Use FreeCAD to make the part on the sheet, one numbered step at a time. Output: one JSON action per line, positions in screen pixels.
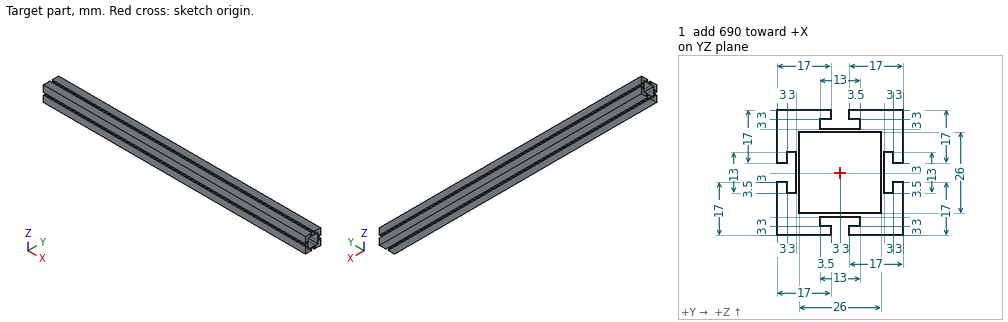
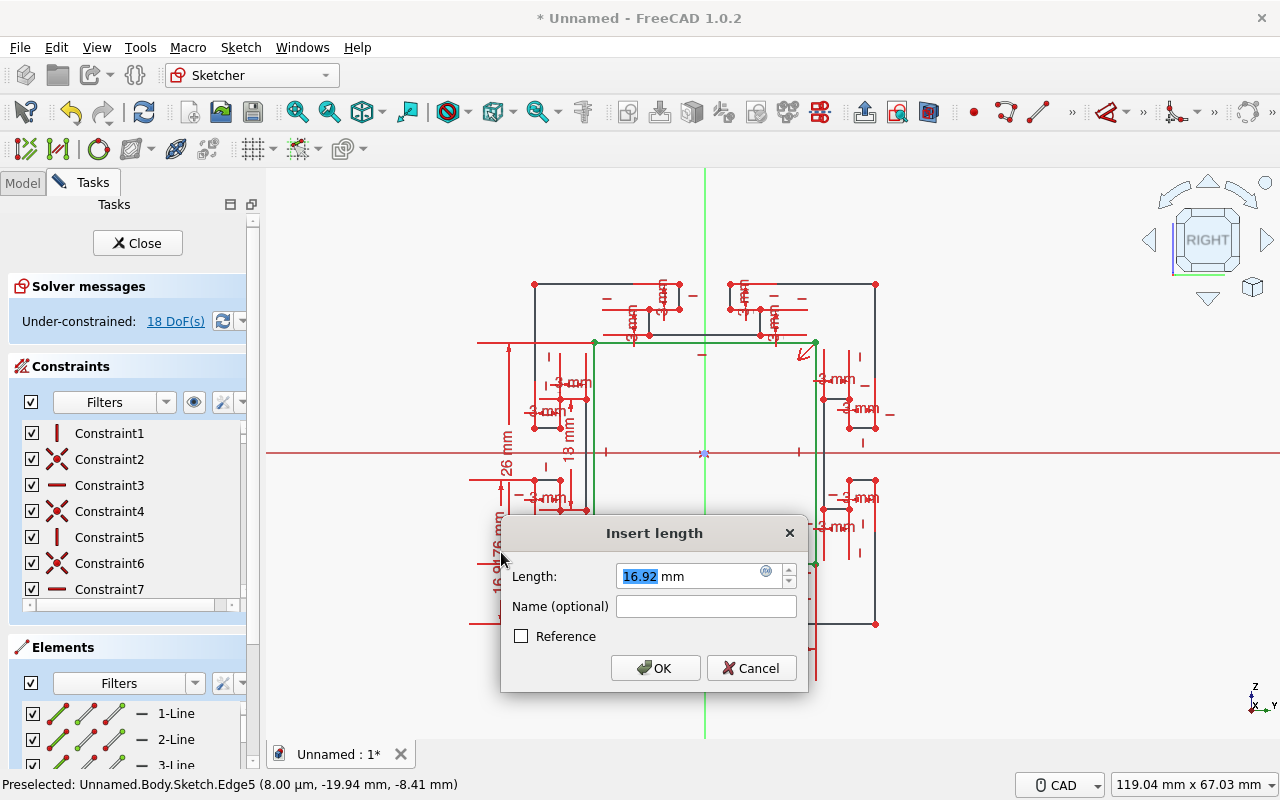
{"action": "type", "text": "17"}
{"action": "key", "text": "Return"}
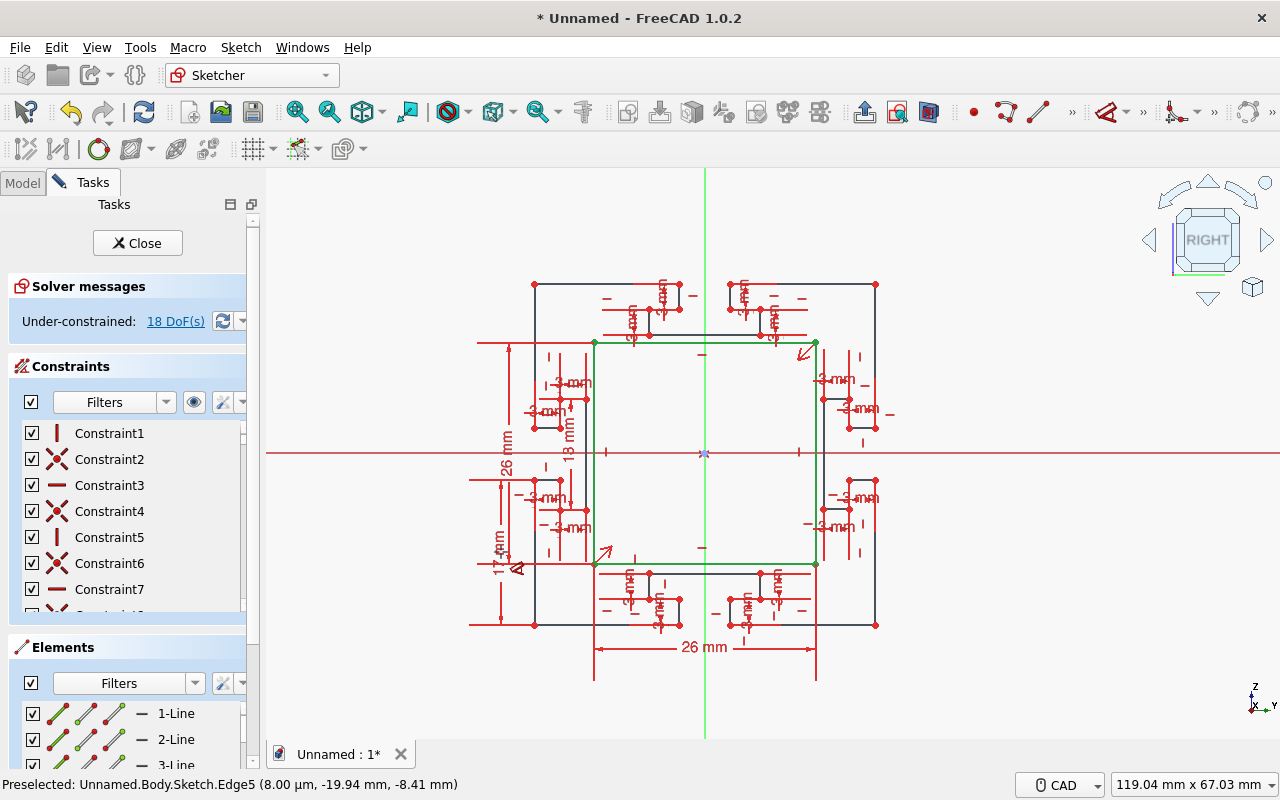
{"action": "left_click", "coordinate": [578, 625]}
{"action": "left_click", "coordinate": [607, 659]}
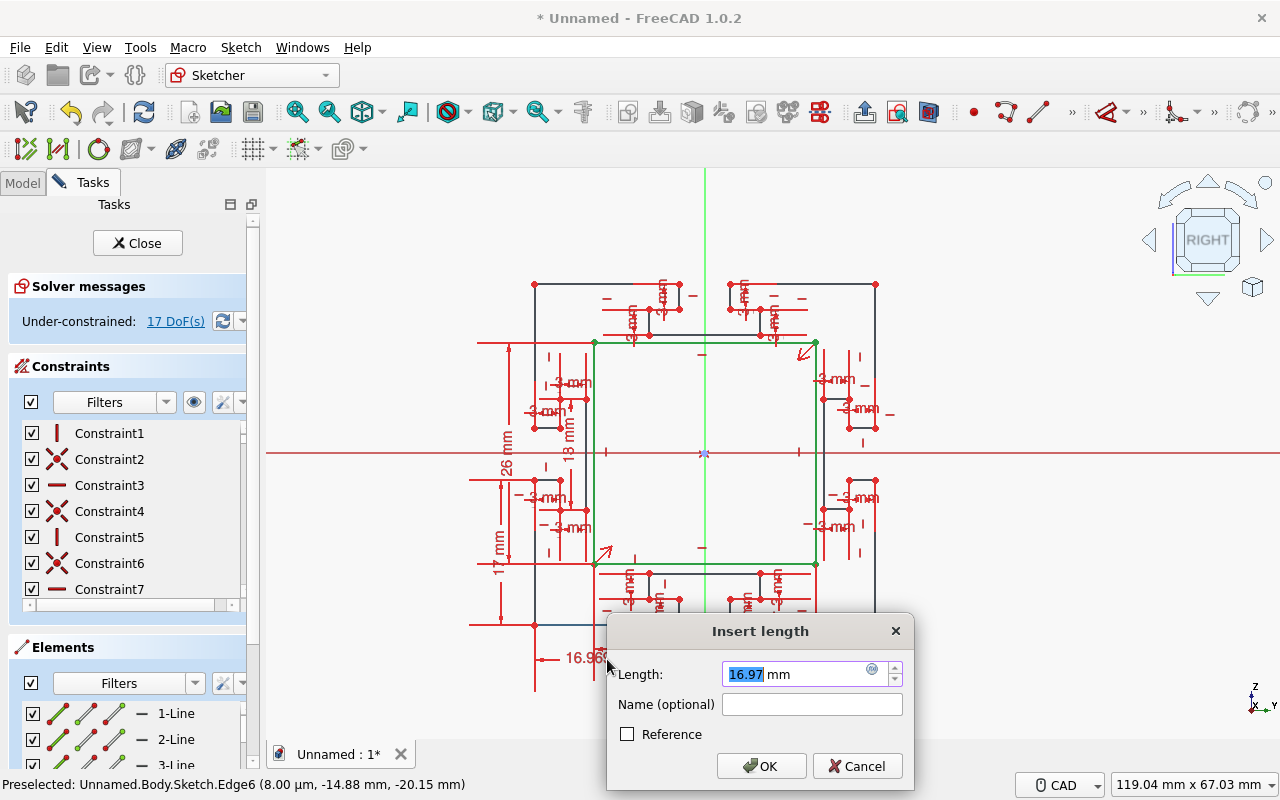
{"action": "type", "text": "17"}
{"action": "key", "text": "Return"}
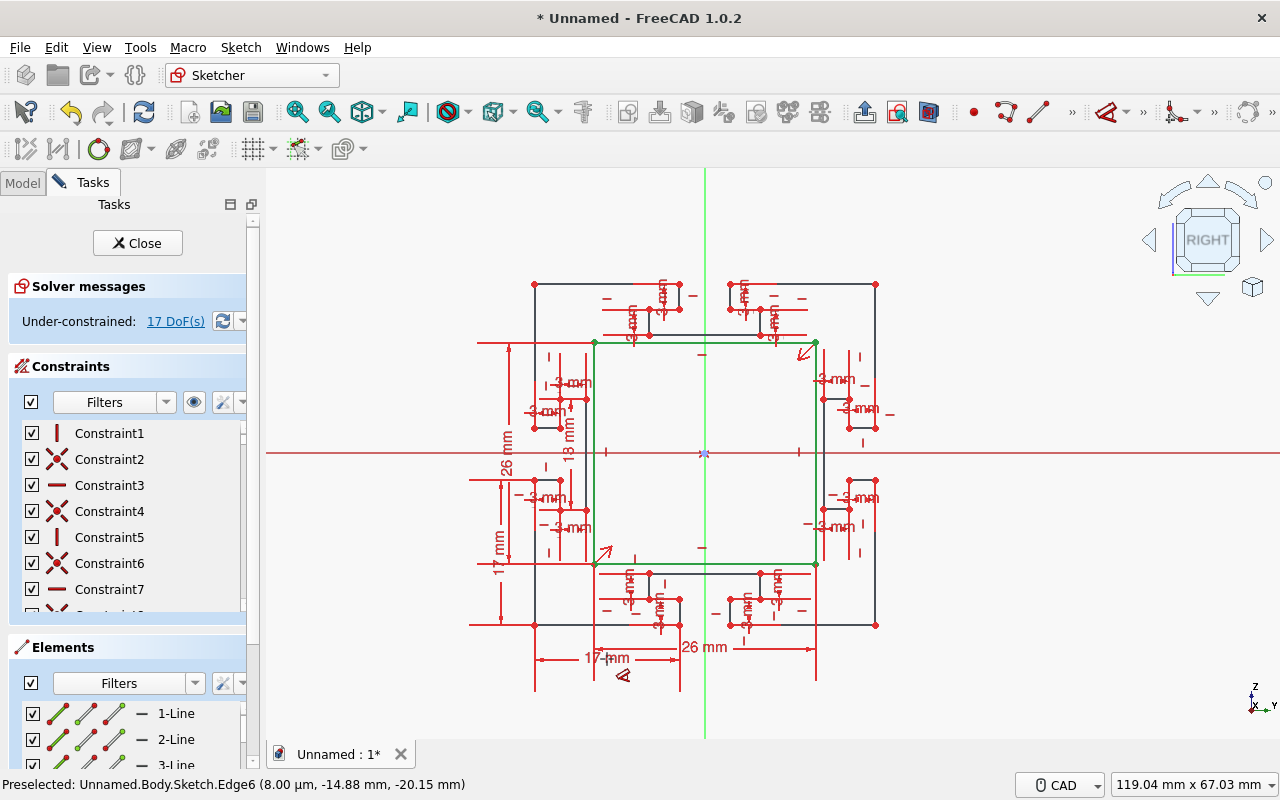
{"action": "scroll", "coordinate": [683, 574], "scroll_direction": "up", "scroll_amount": 2}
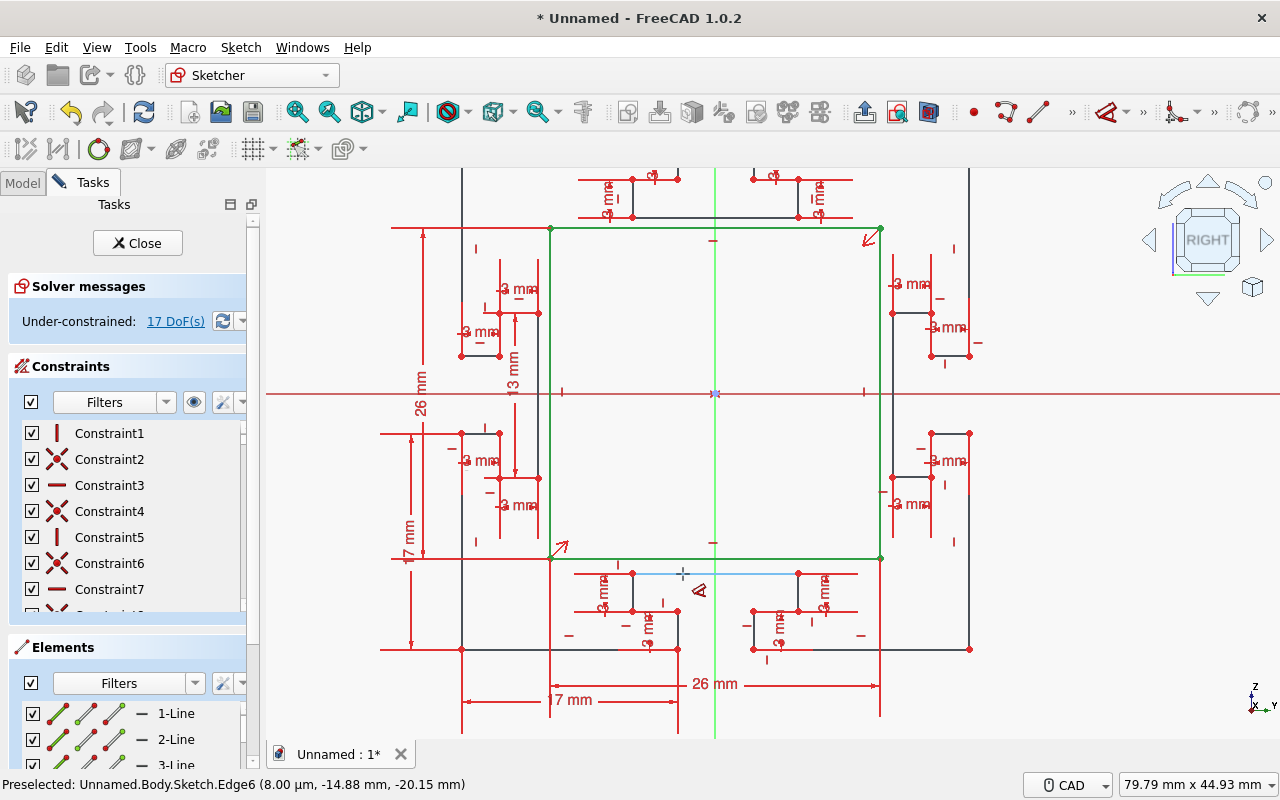
{"action": "left_click", "coordinate": [682, 574]}
{"action": "left_click", "coordinate": [677, 540]}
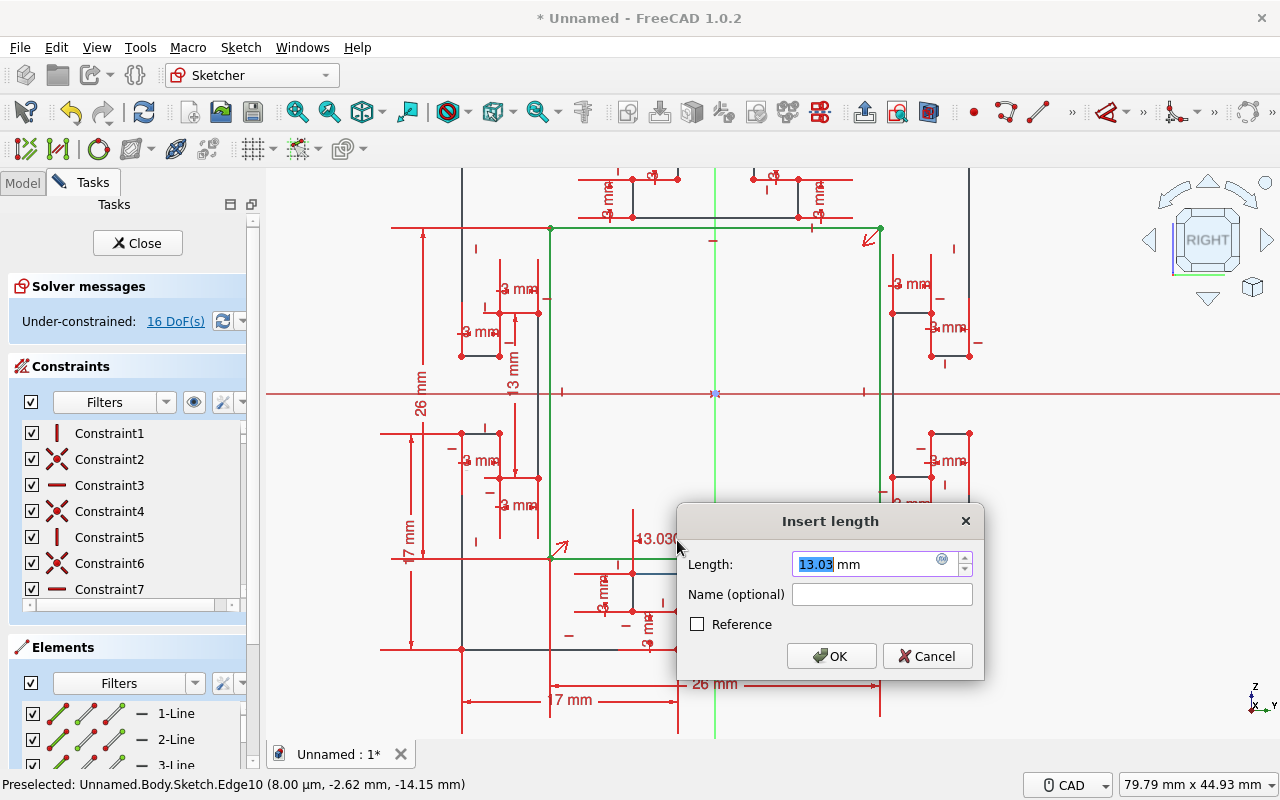
{"action": "type", "text": "13"}
{"action": "key", "text": "Return"}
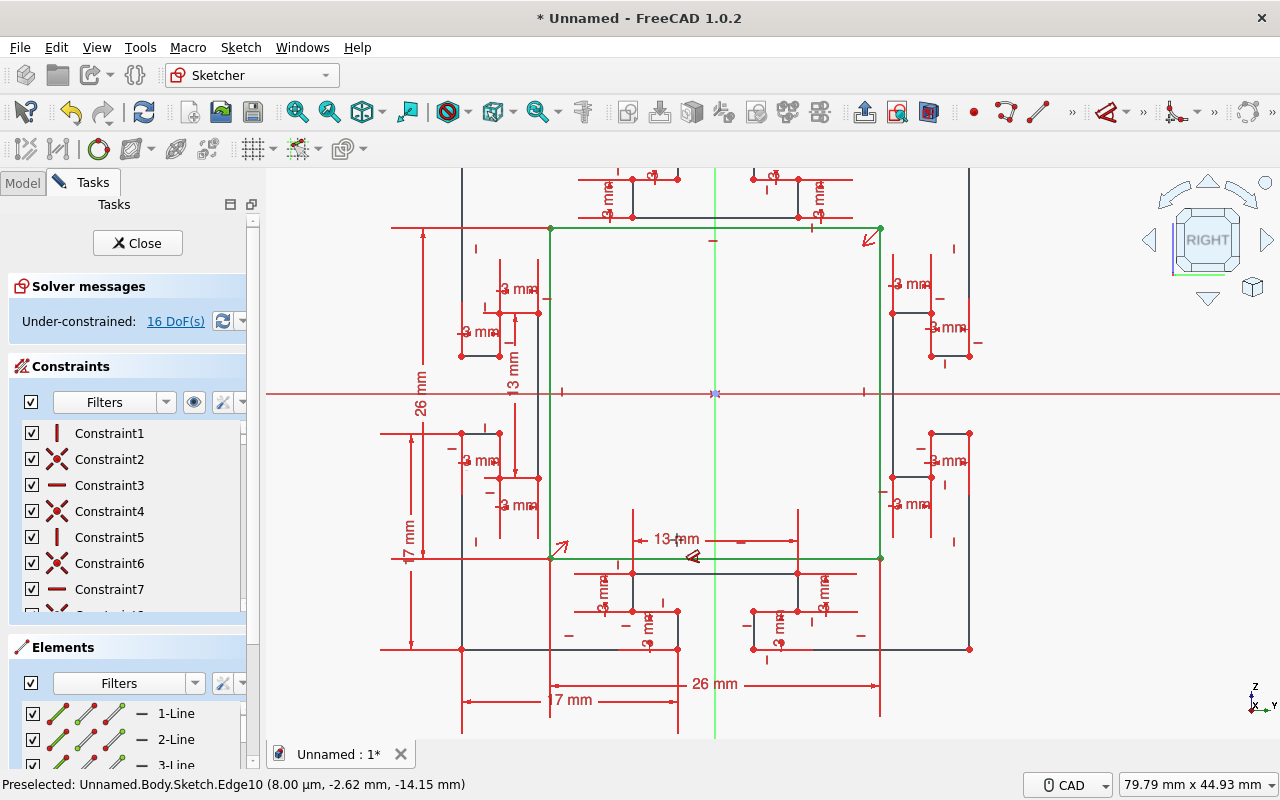
{"action": "left_click", "coordinate": [818, 650]}
{"action": "left_click", "coordinate": [861, 684]}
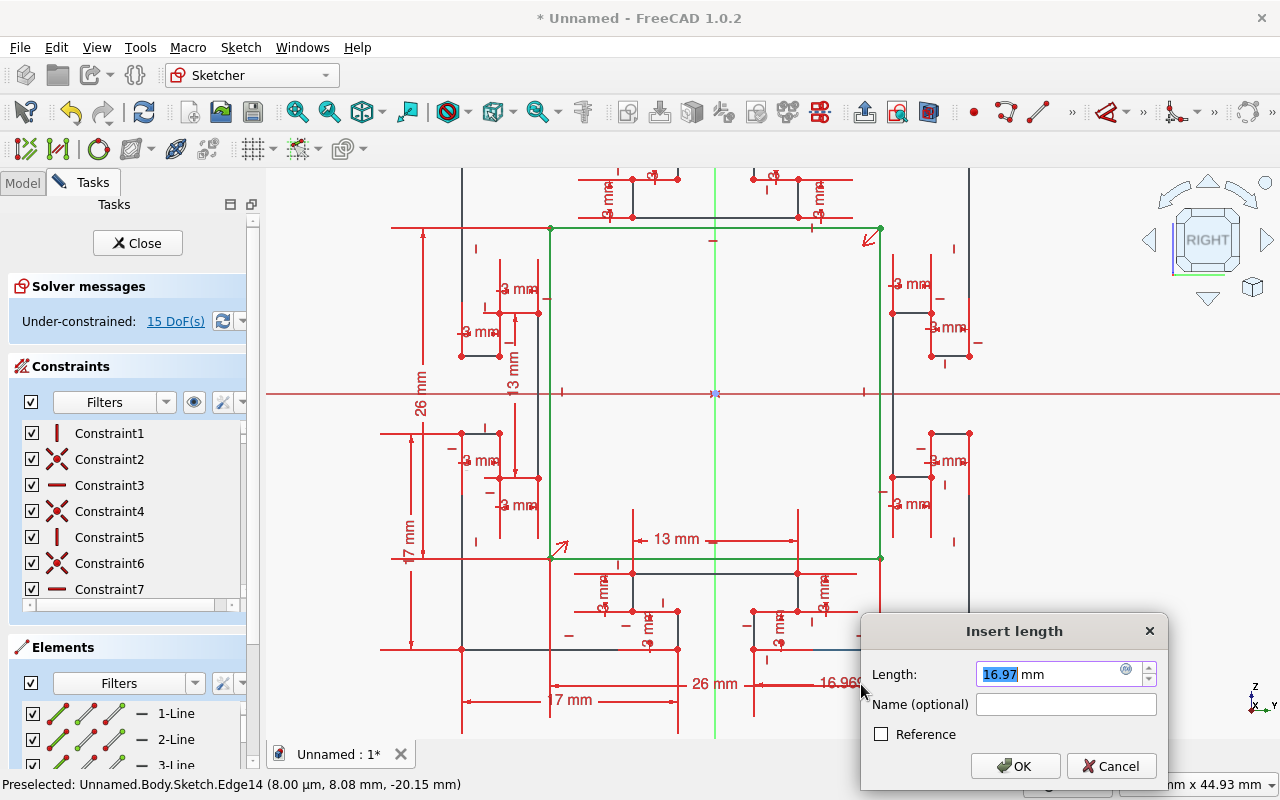
{"action": "type", "text": "17"}
{"action": "key", "text": "Return"}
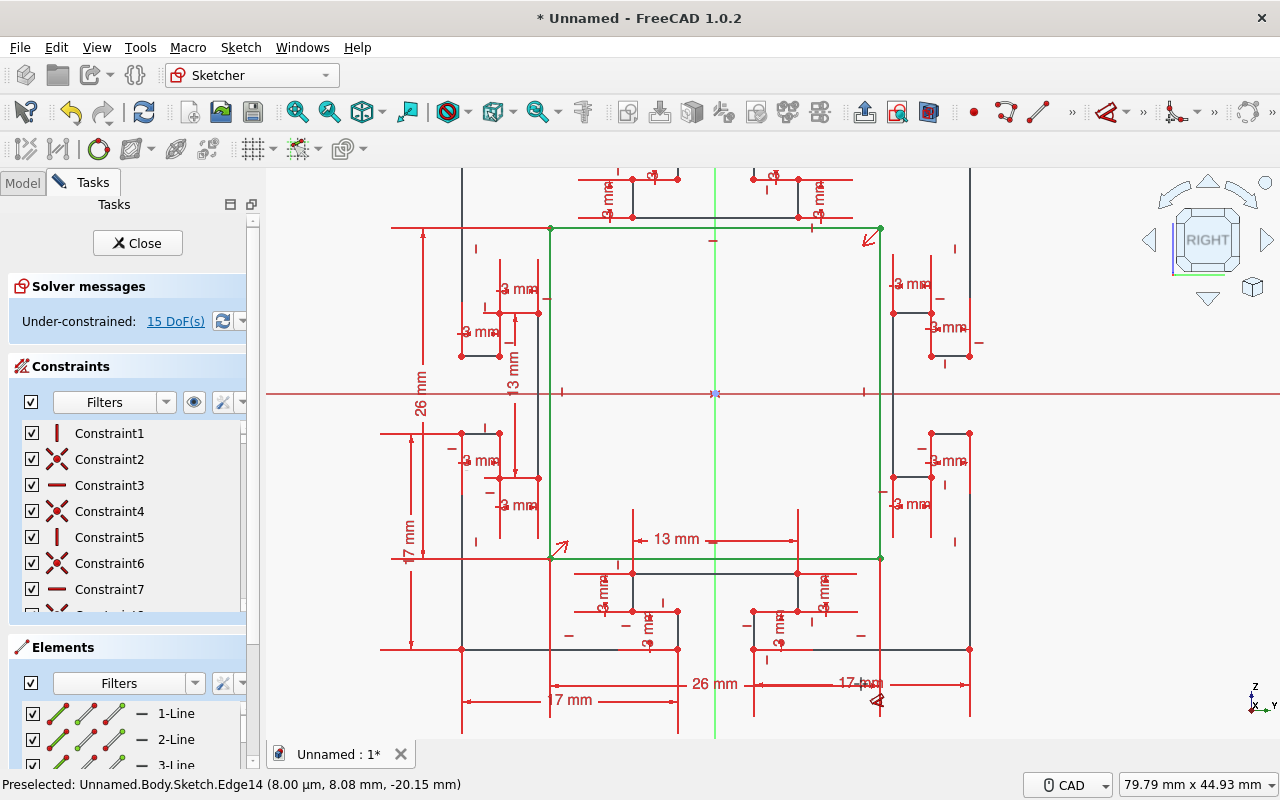
{"action": "left_click", "coordinate": [970, 585]}
{"action": "left_click", "coordinate": [1004, 542]}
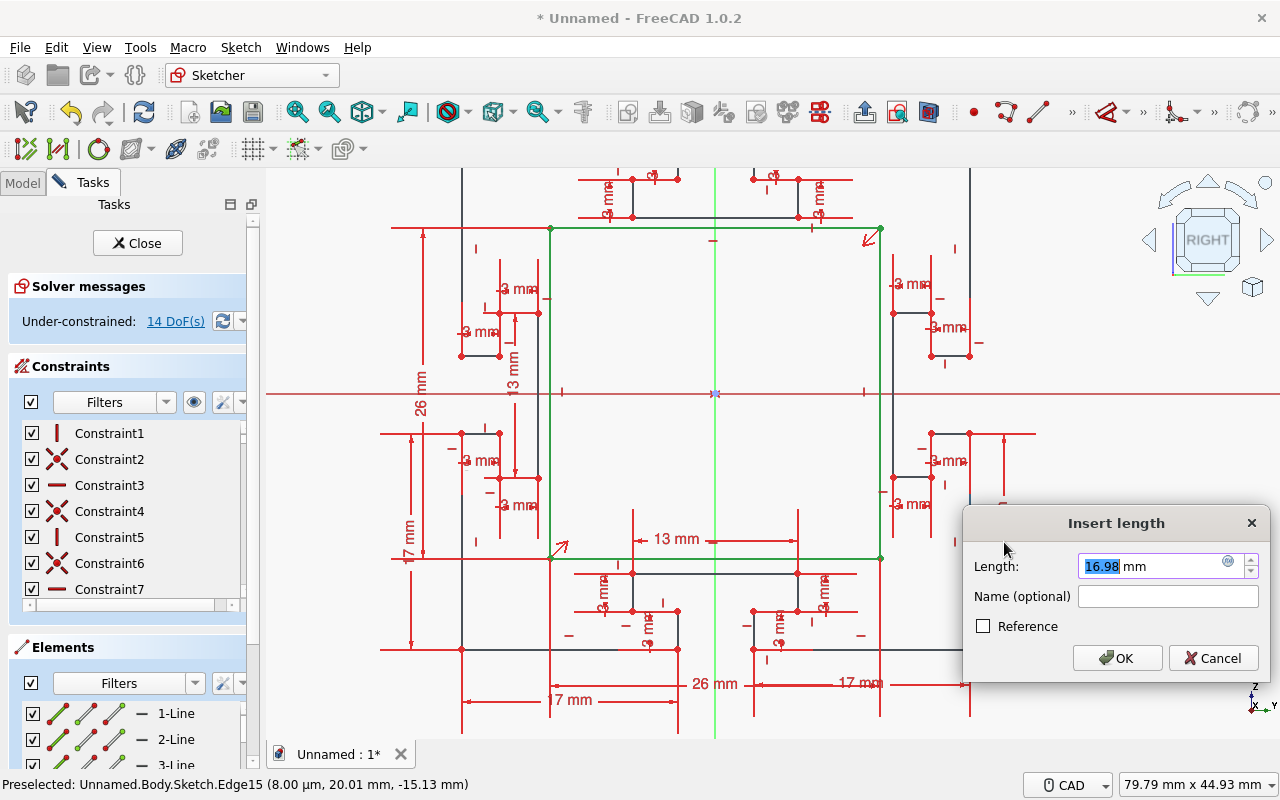
{"action": "type", "text": "17"}
{"action": "key", "text": "Return"}